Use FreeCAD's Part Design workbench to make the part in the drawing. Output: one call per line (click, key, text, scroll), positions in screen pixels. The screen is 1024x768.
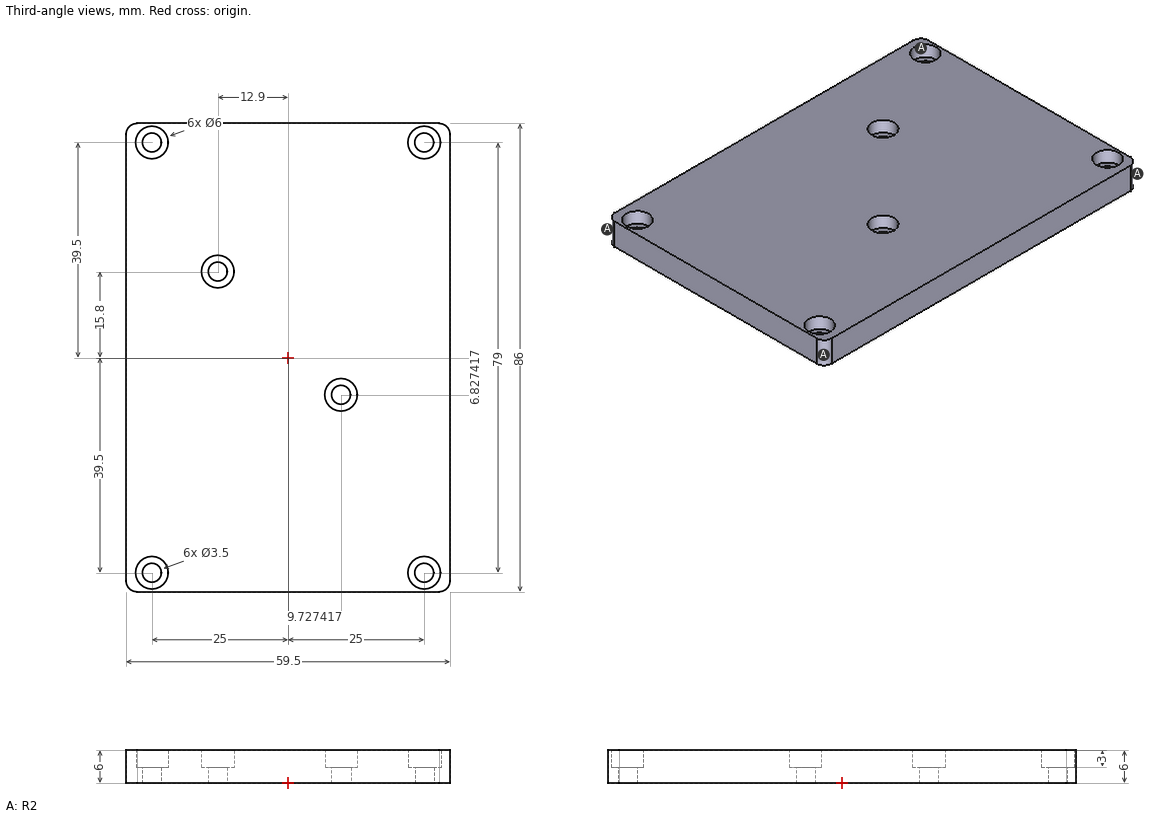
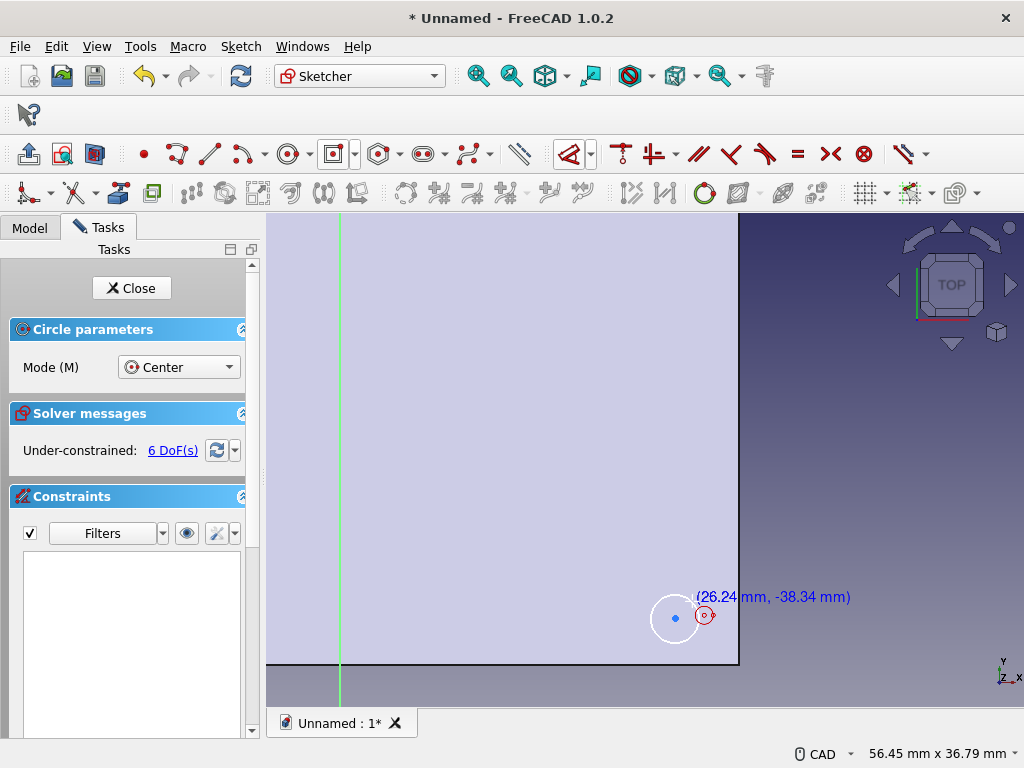
scroll(679, 621, down, 6)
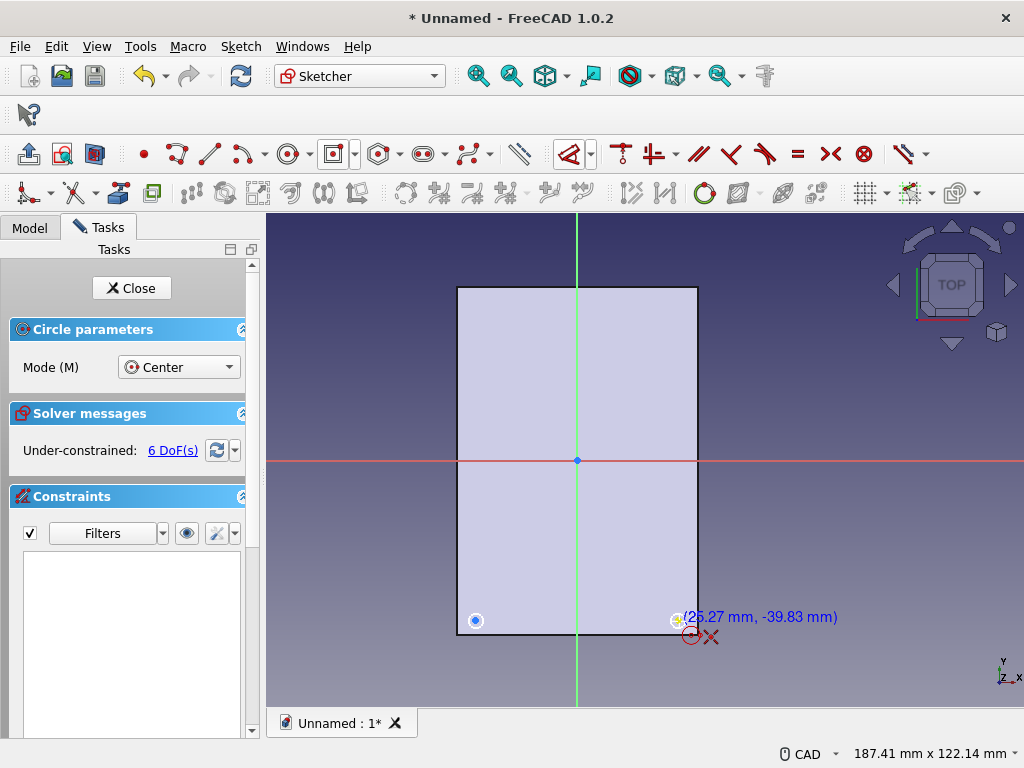
scroll(678, 301, up, 6)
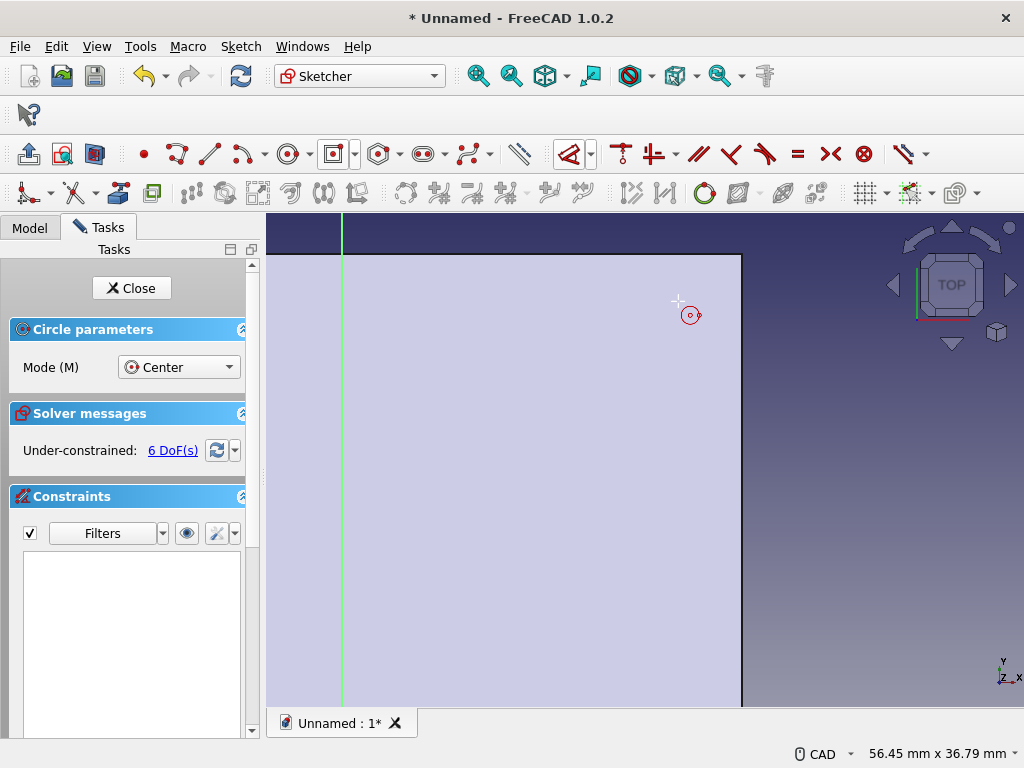
click(678, 301)
click(694, 284)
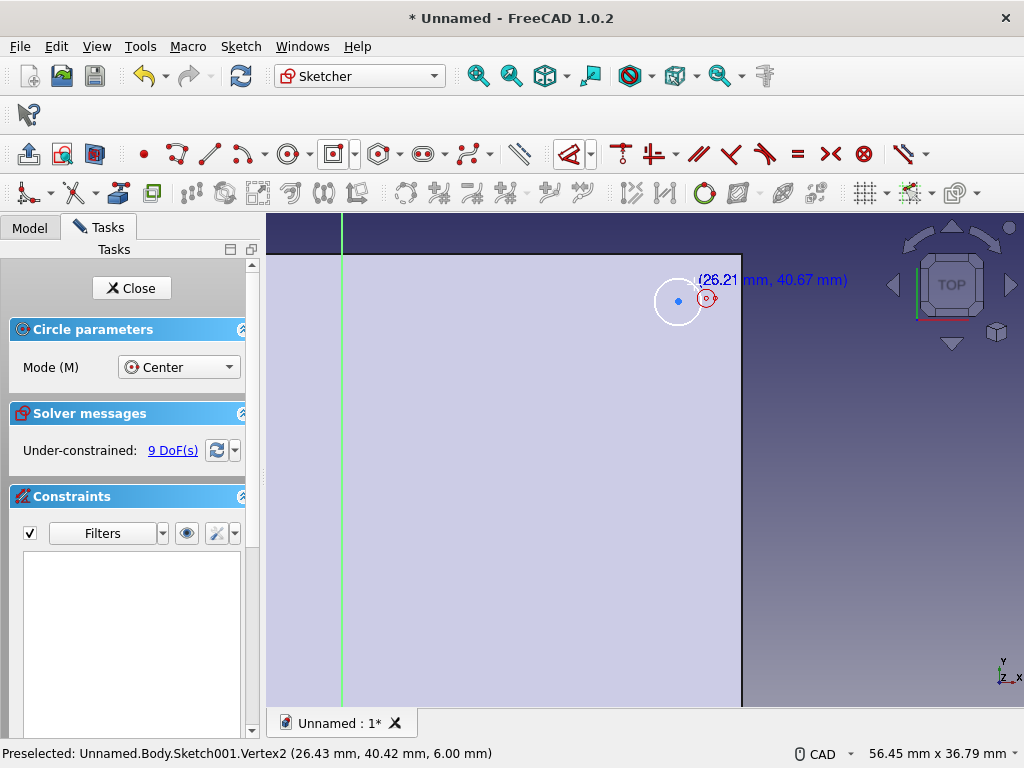
scroll(678, 300, down, 6)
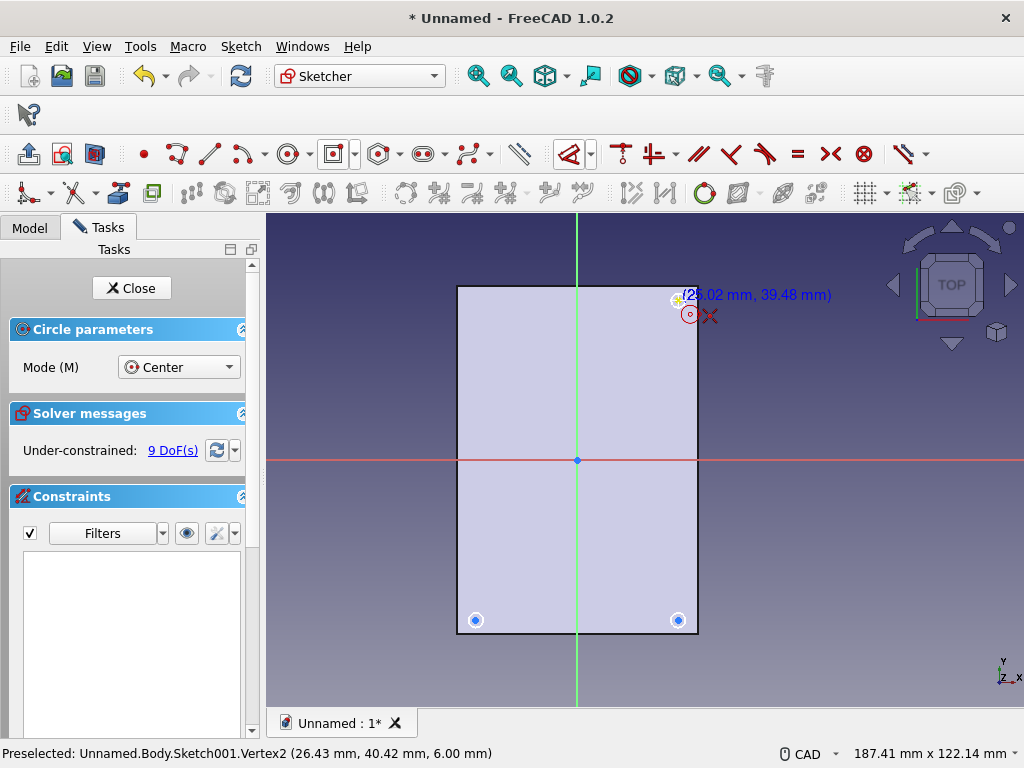
scroll(476, 300, up, 6)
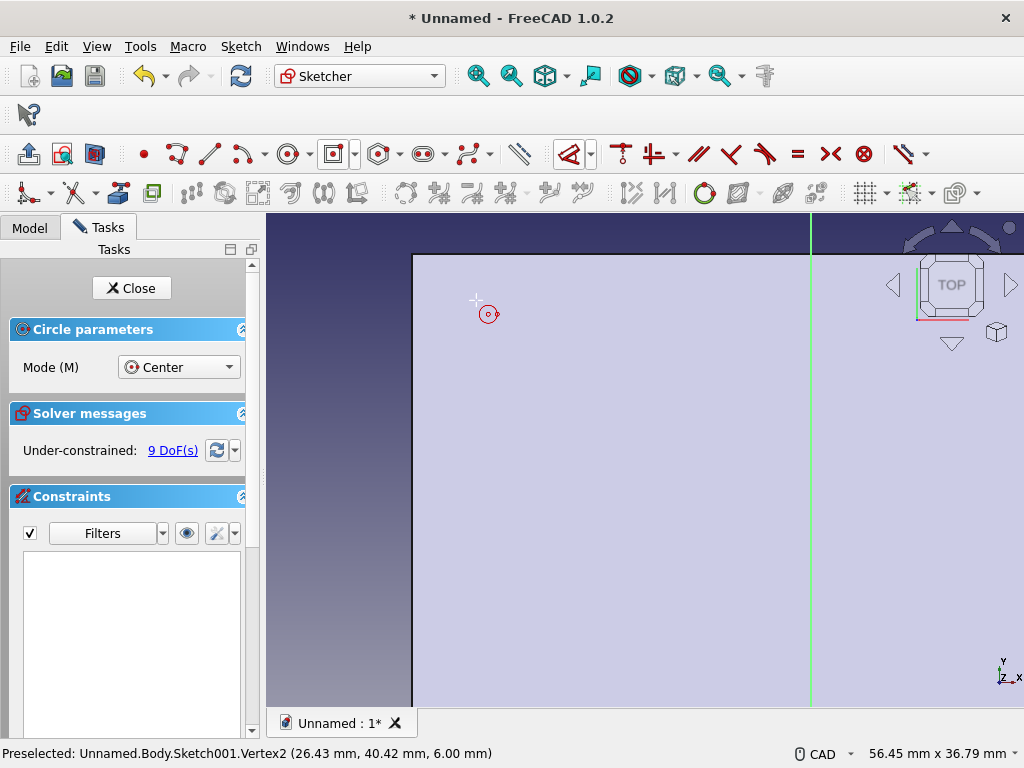
click(476, 301)
click(492, 284)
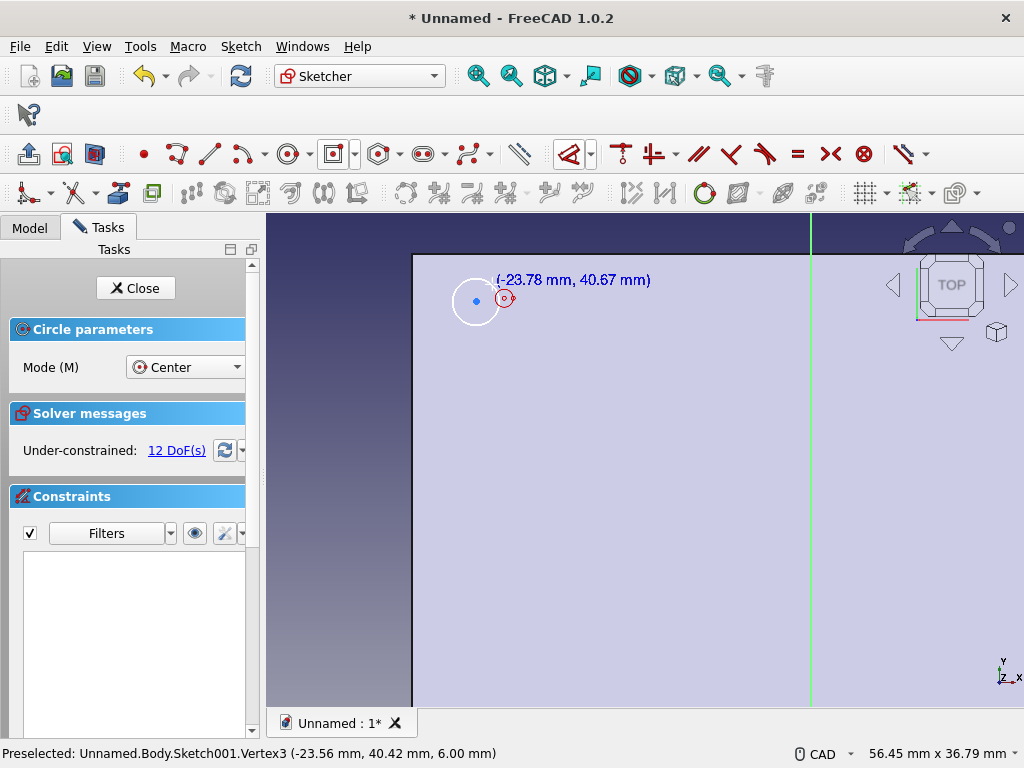
click(638, 619)
click(655, 602)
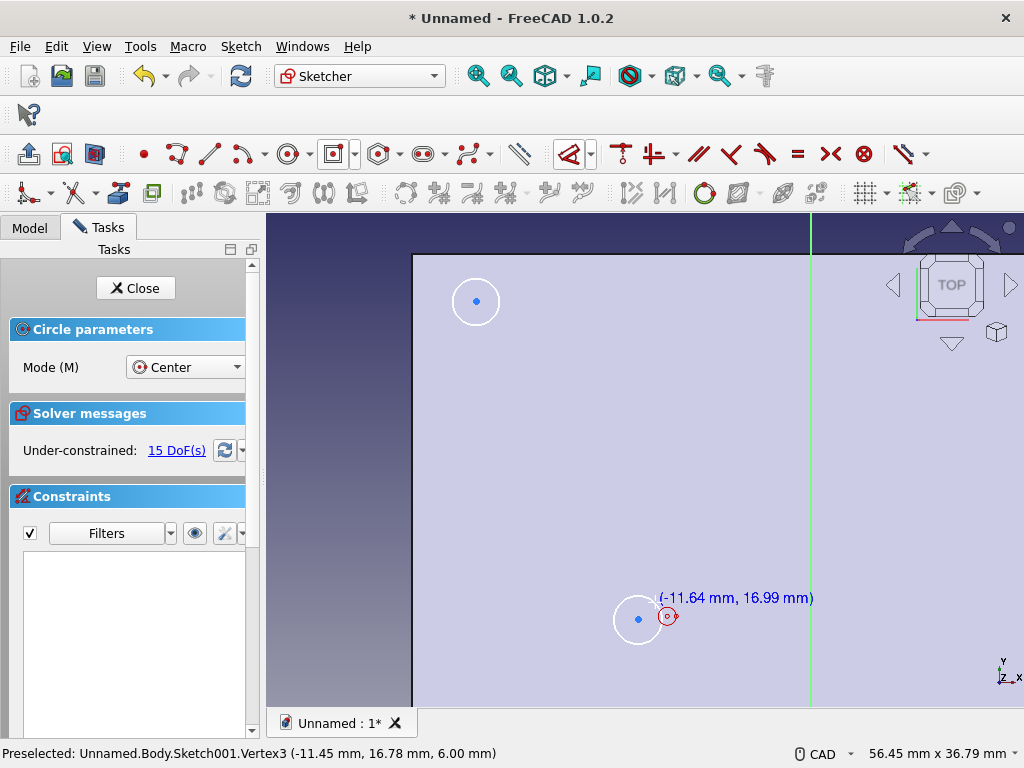
scroll(475, 300, down, 6)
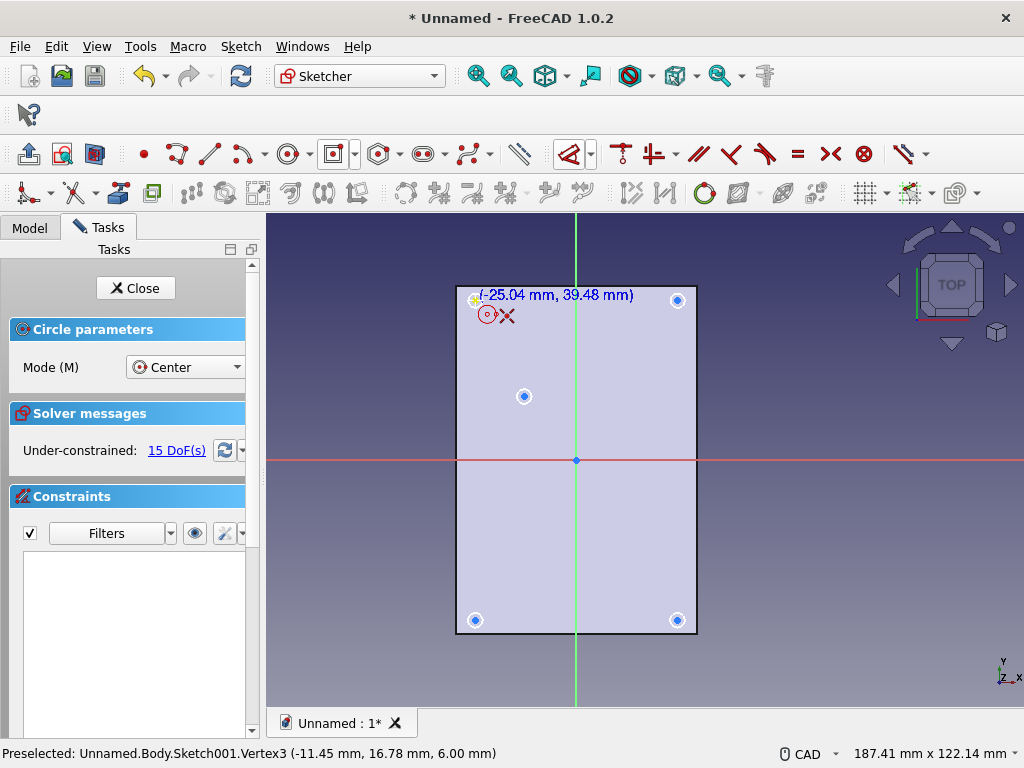
scroll(616, 488, up, 6)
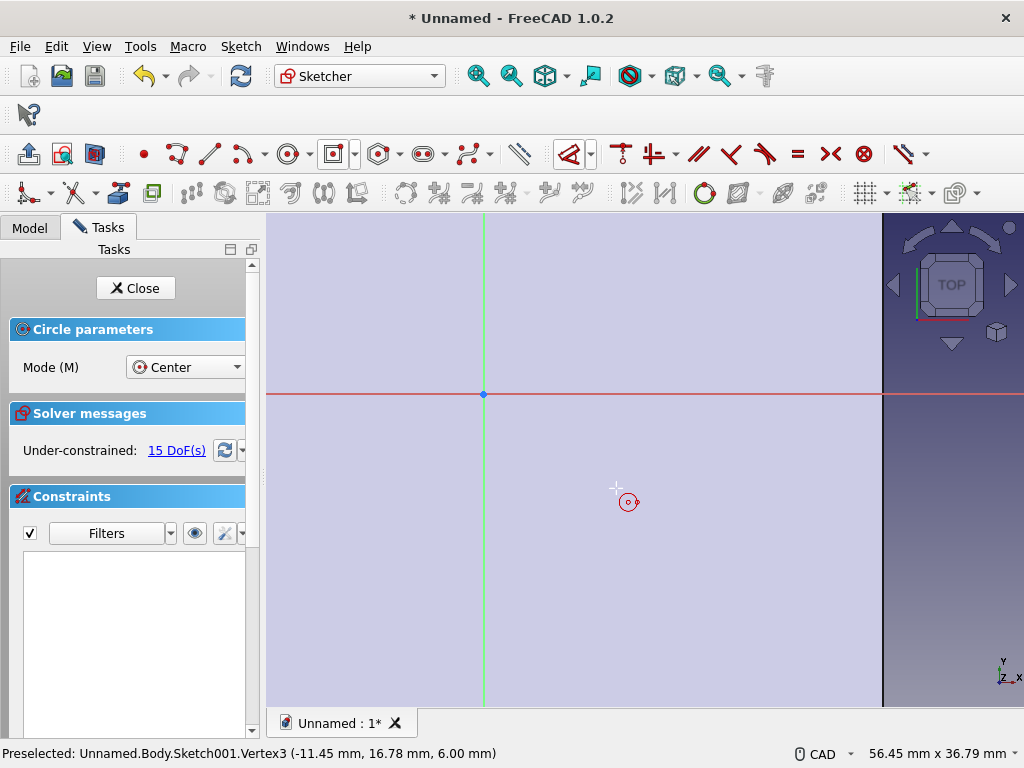
click(614, 486)
click(631, 469)
key(Escape)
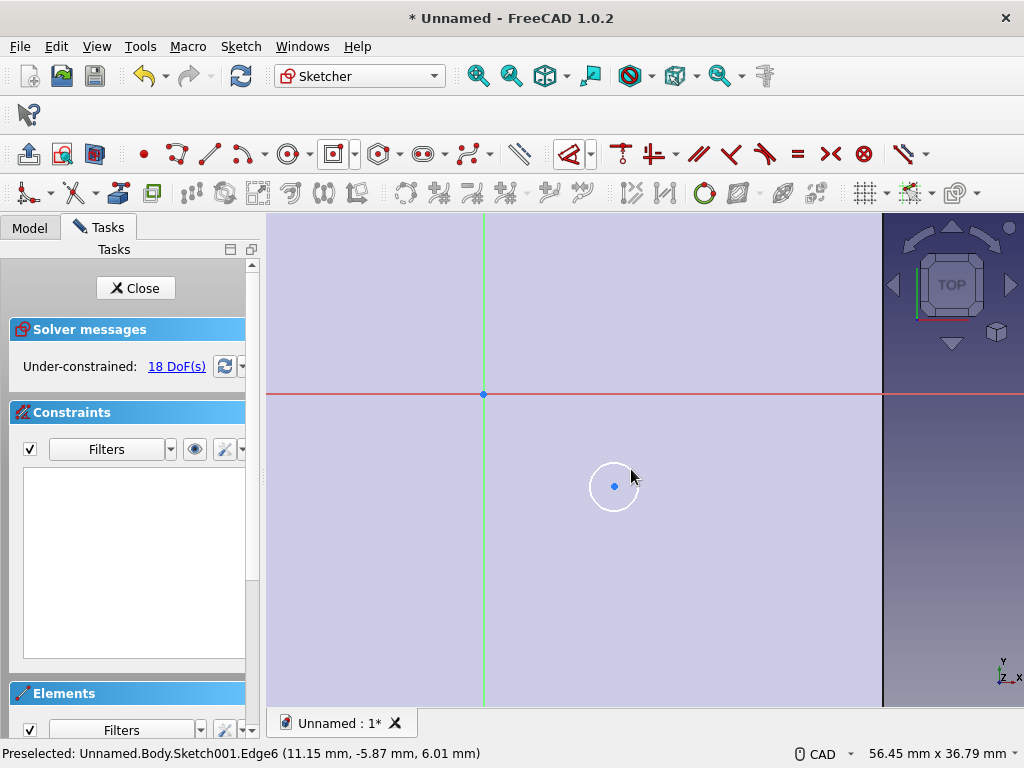
scroll(616, 488, down, 6)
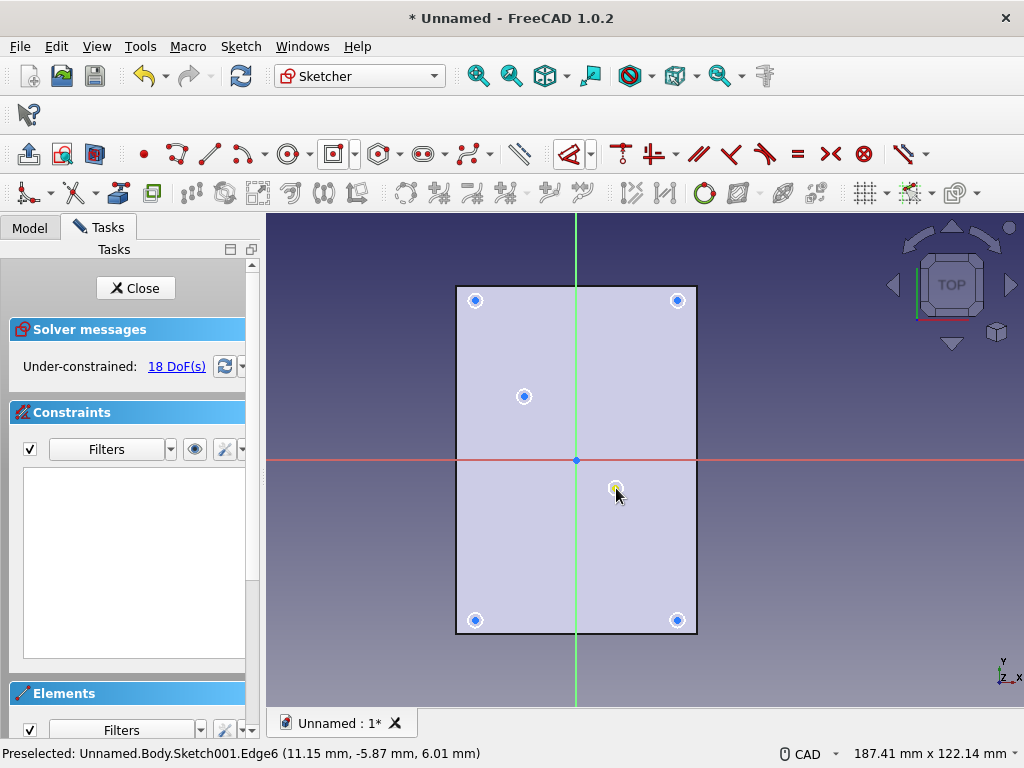
scroll(480, 615, up, 4)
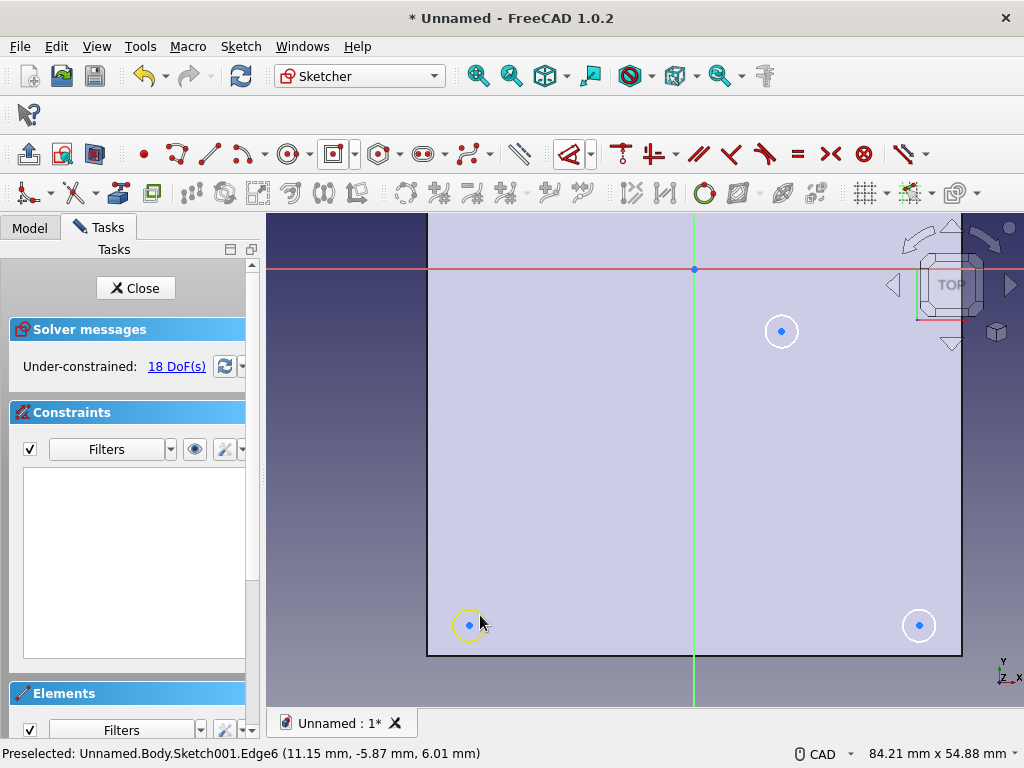
click(481, 614)